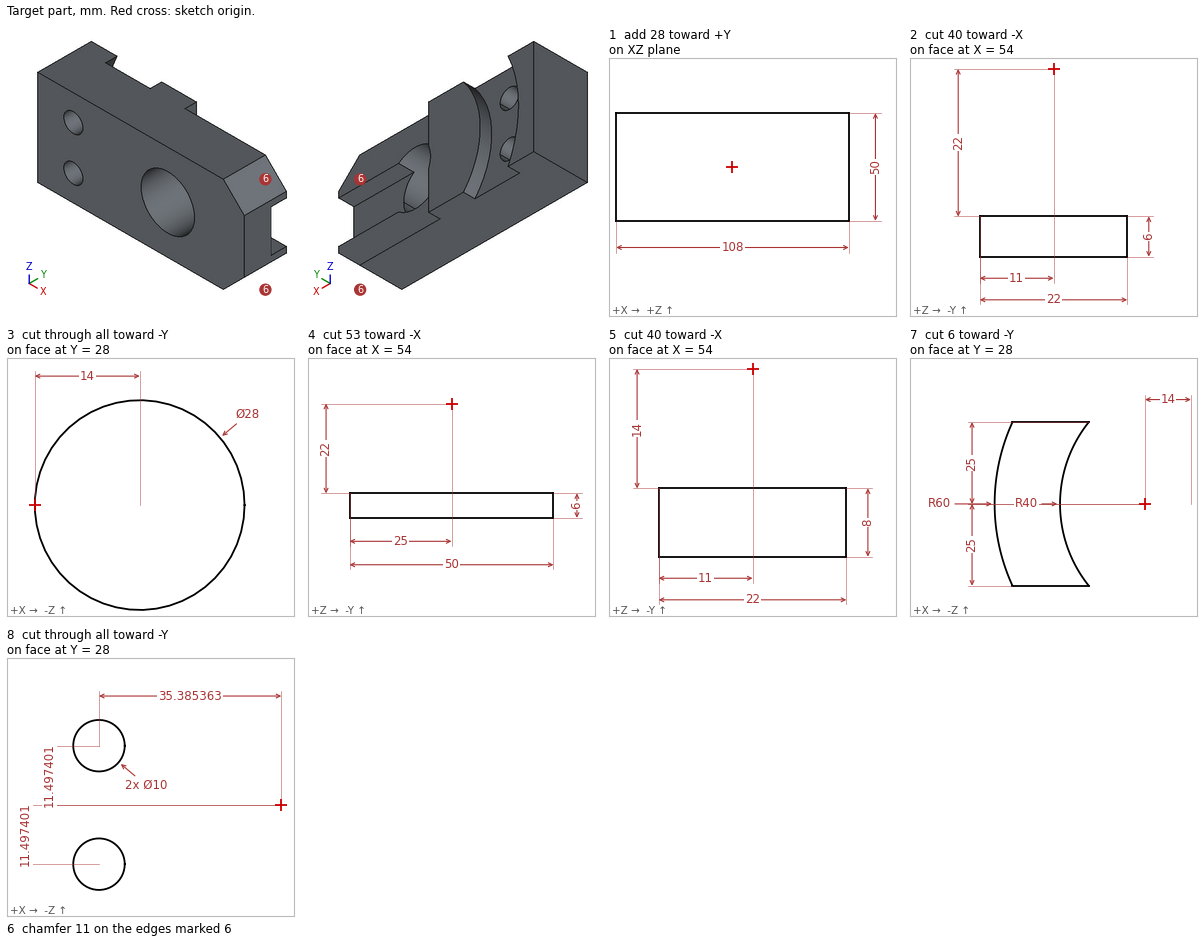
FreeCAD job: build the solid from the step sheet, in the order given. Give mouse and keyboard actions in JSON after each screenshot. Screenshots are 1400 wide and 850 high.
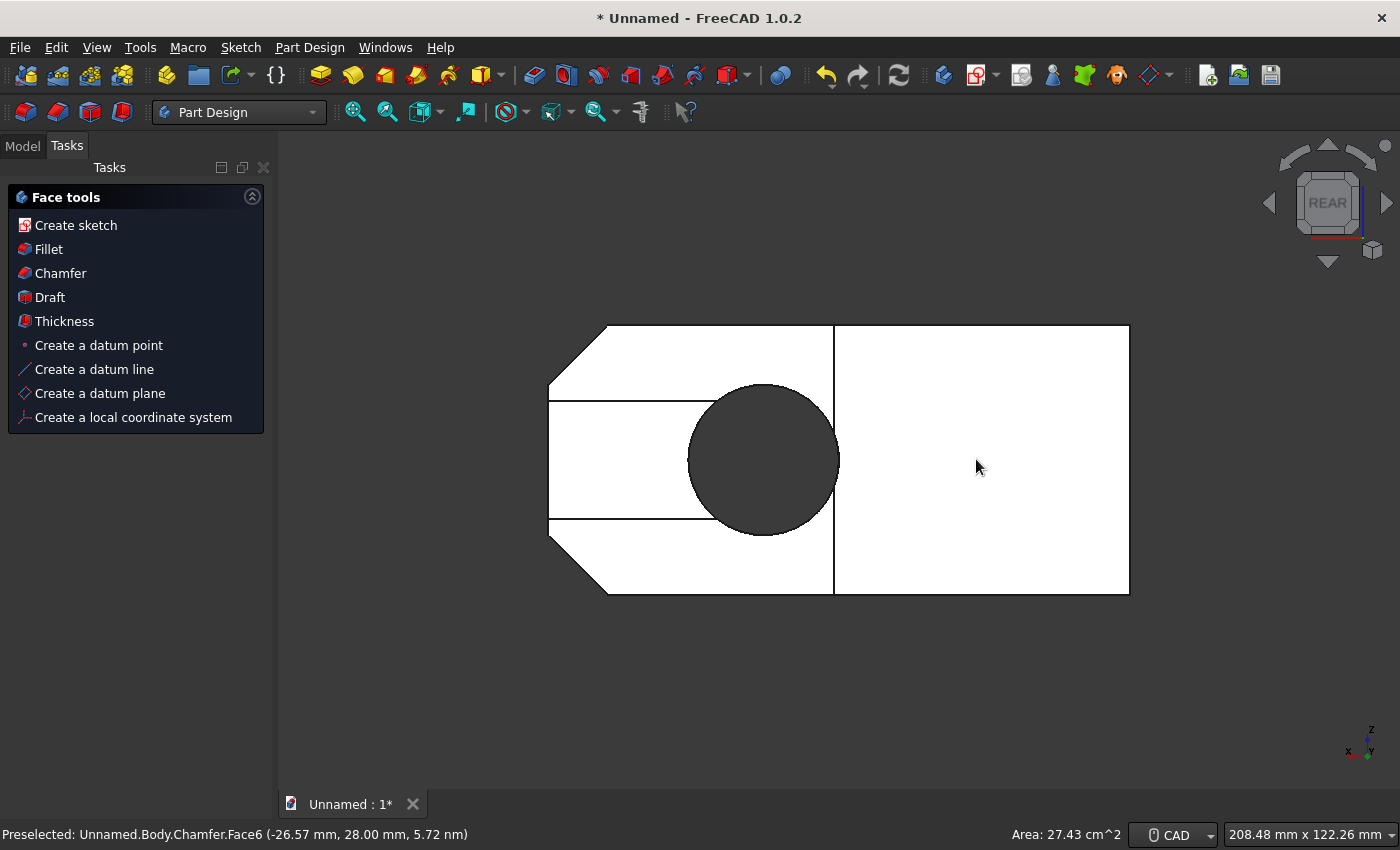
{"action": "left_click", "coordinate": [976, 76]}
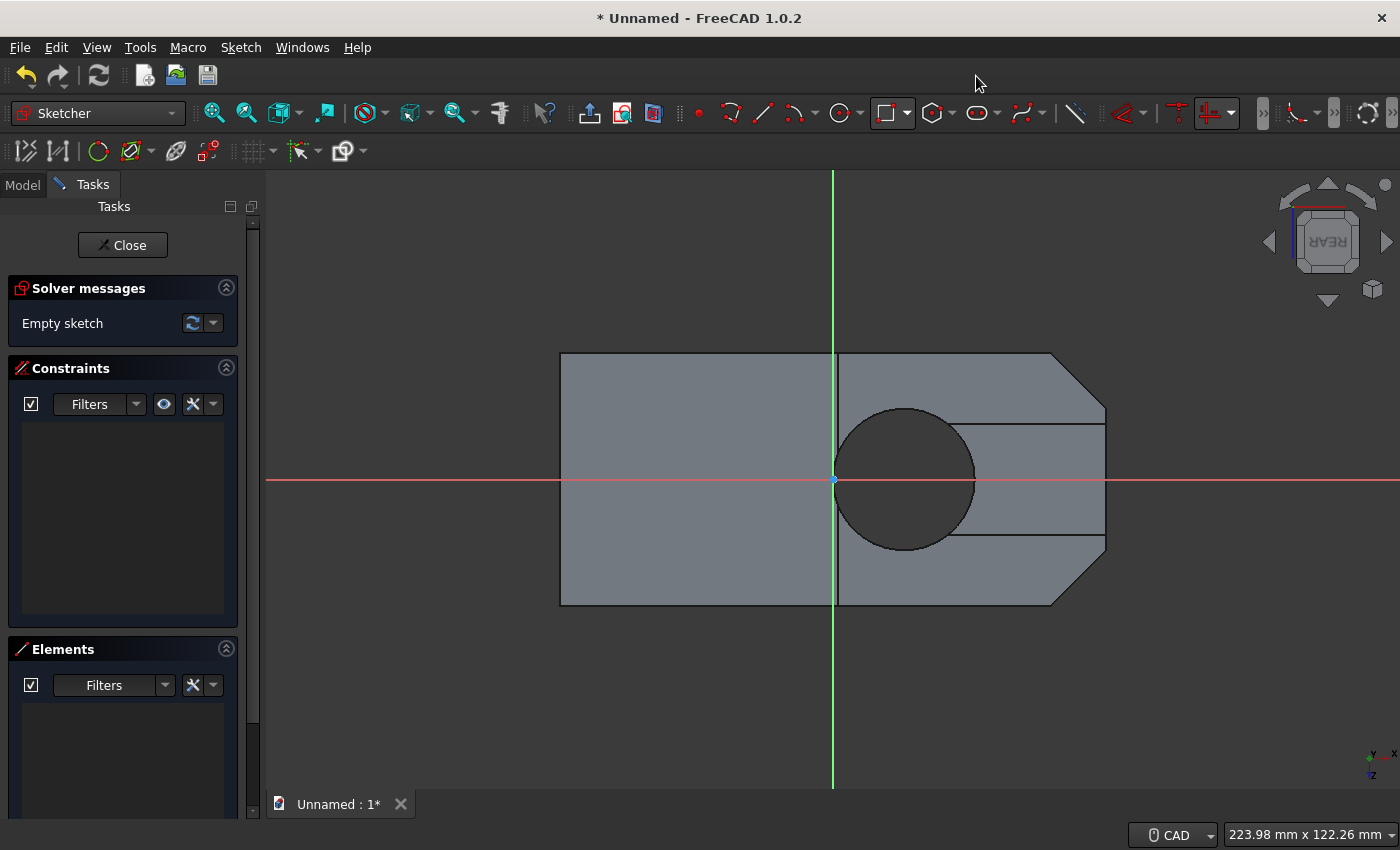
{"action": "scroll", "coordinate": [619, 479], "scroll_direction": "up", "scroll_amount": 2}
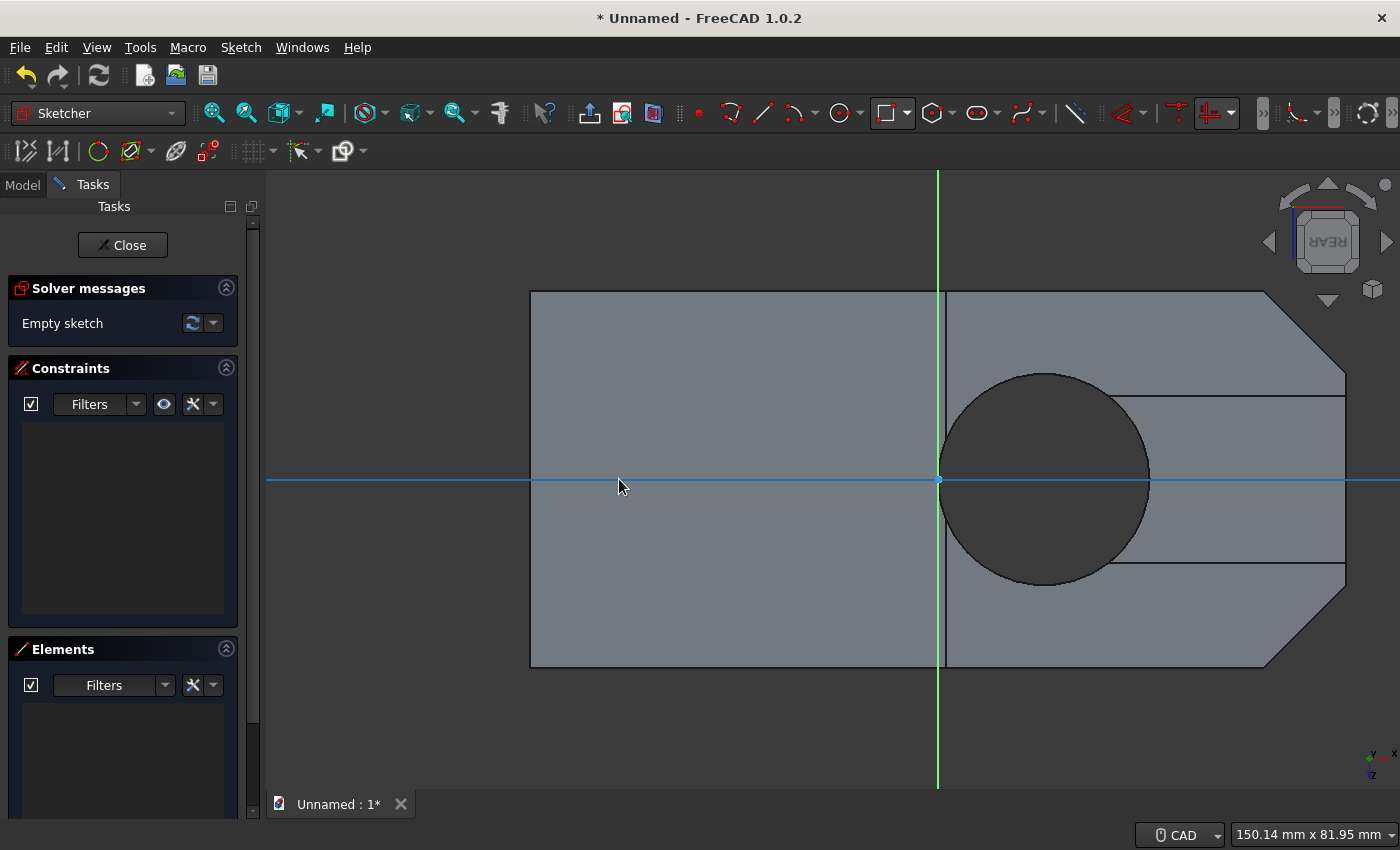
{"action": "key", "text": "g l"}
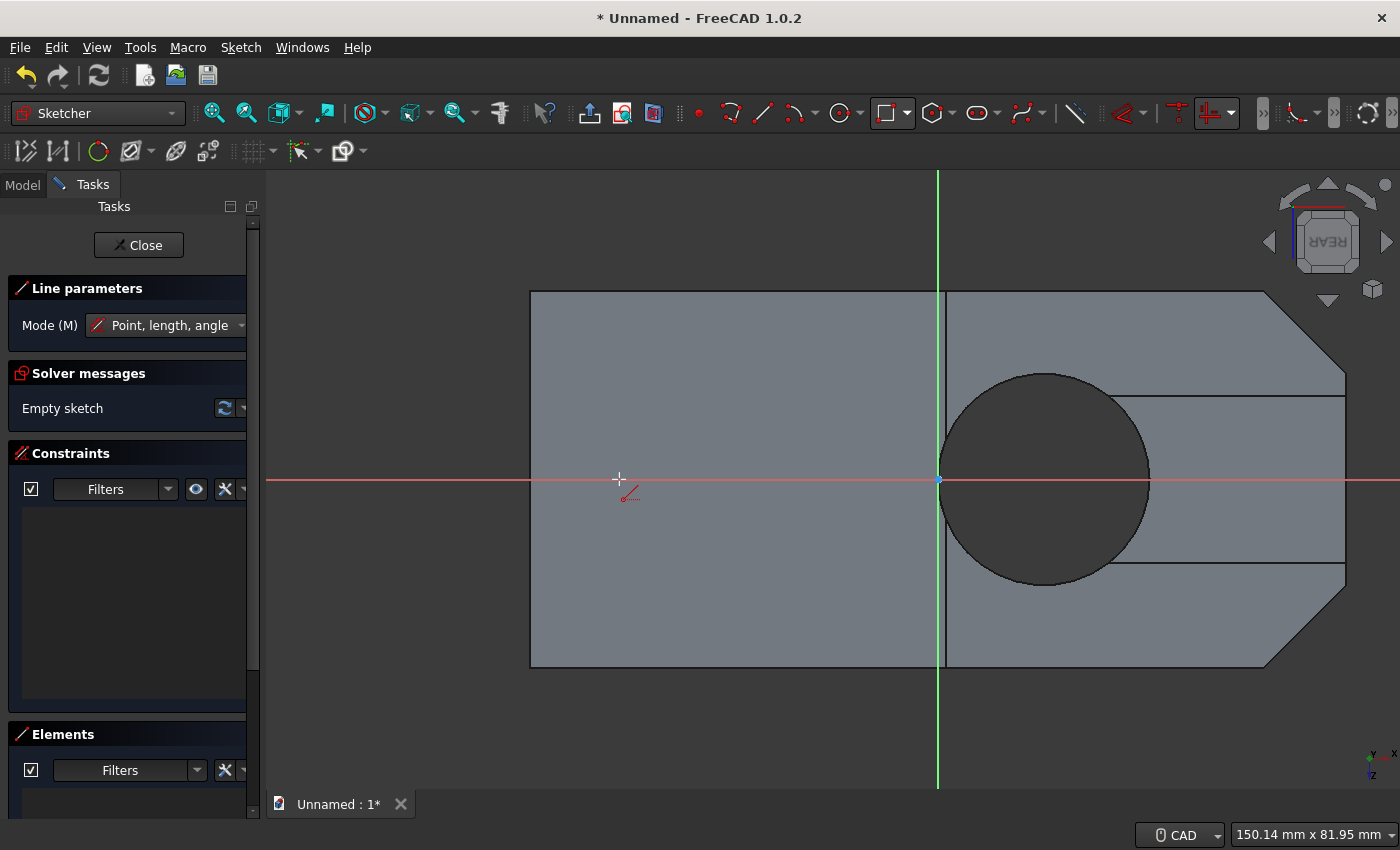
{"action": "left_click", "coordinate": [632, 668]}
{"action": "left_click", "coordinate": [808, 668]}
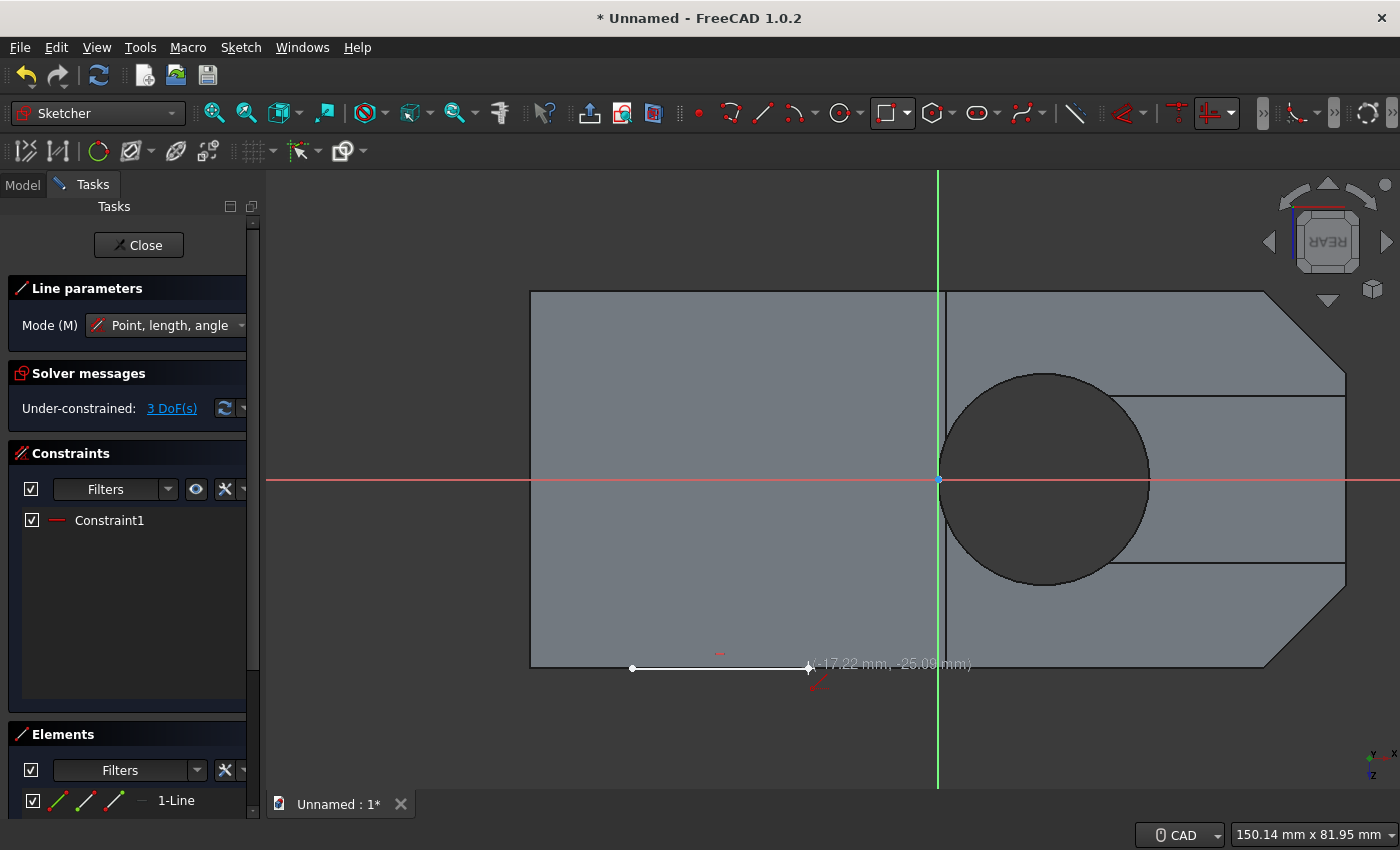
{"action": "left_click", "coordinate": [808, 291]}
{"action": "left_click", "coordinate": [632, 291]}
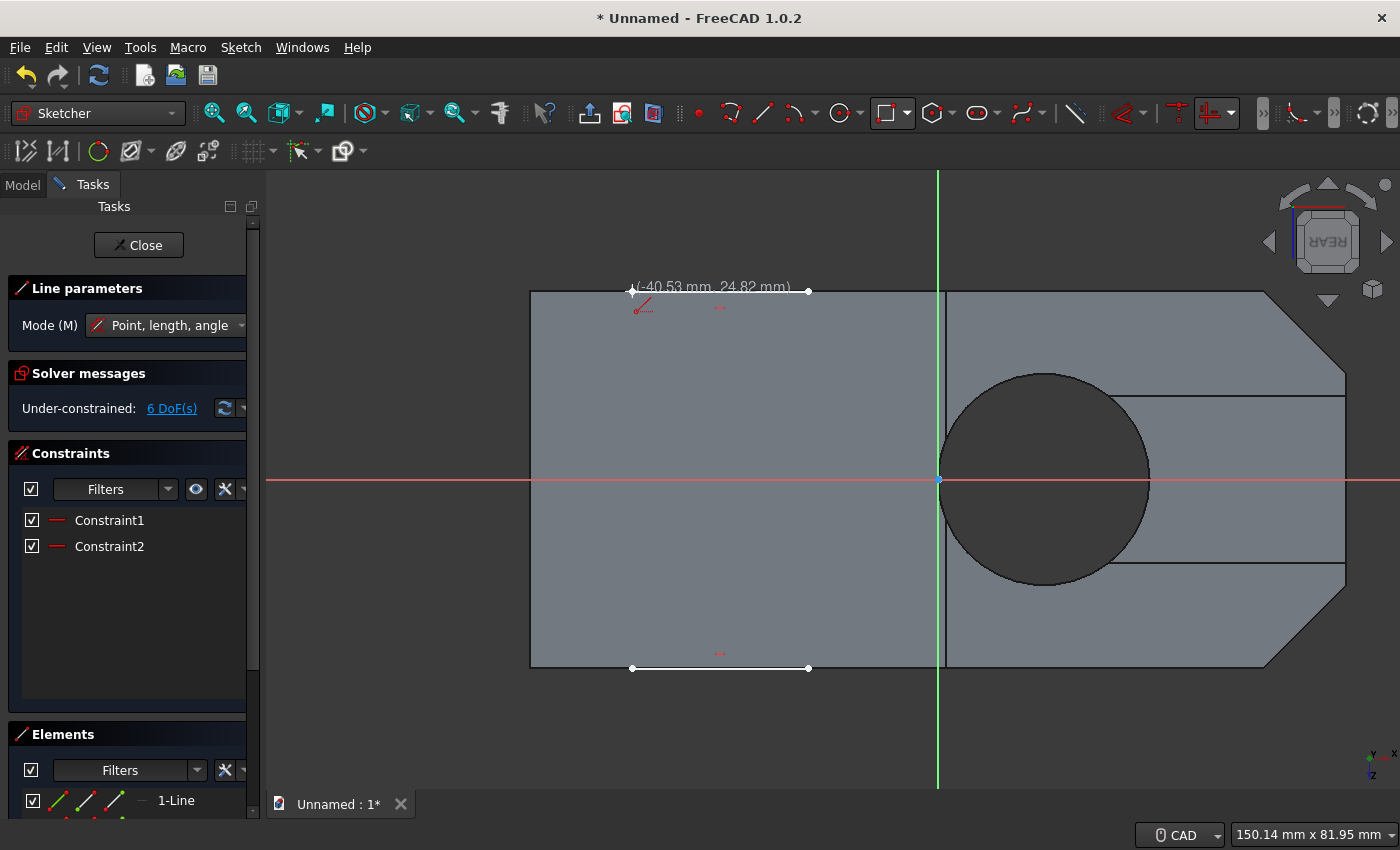
{"action": "key", "text": "g 3 a"}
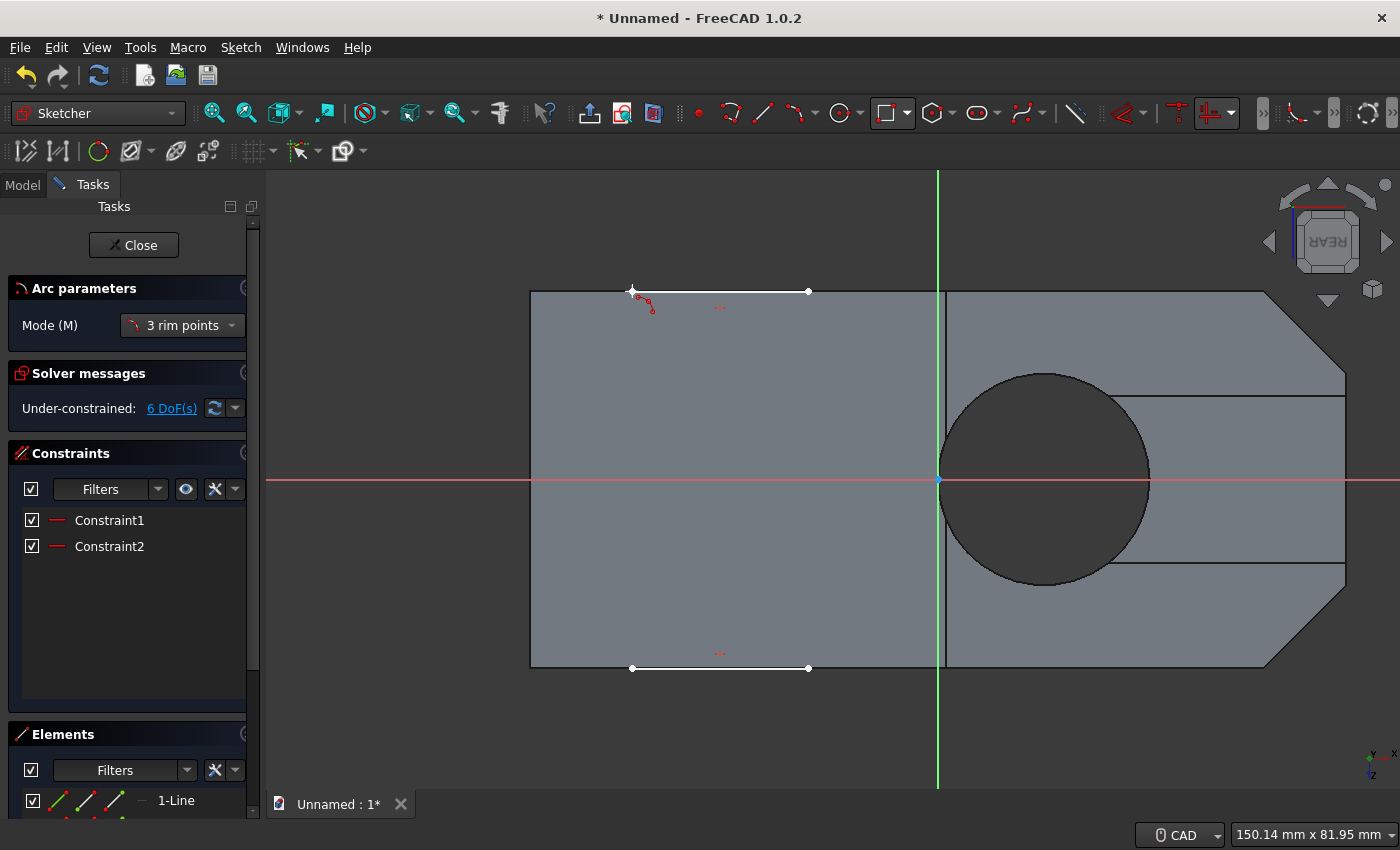
{"action": "left_click", "coordinate": [808, 669]}
{"action": "left_click", "coordinate": [808, 292]}
{"action": "left_click", "coordinate": [744, 439]}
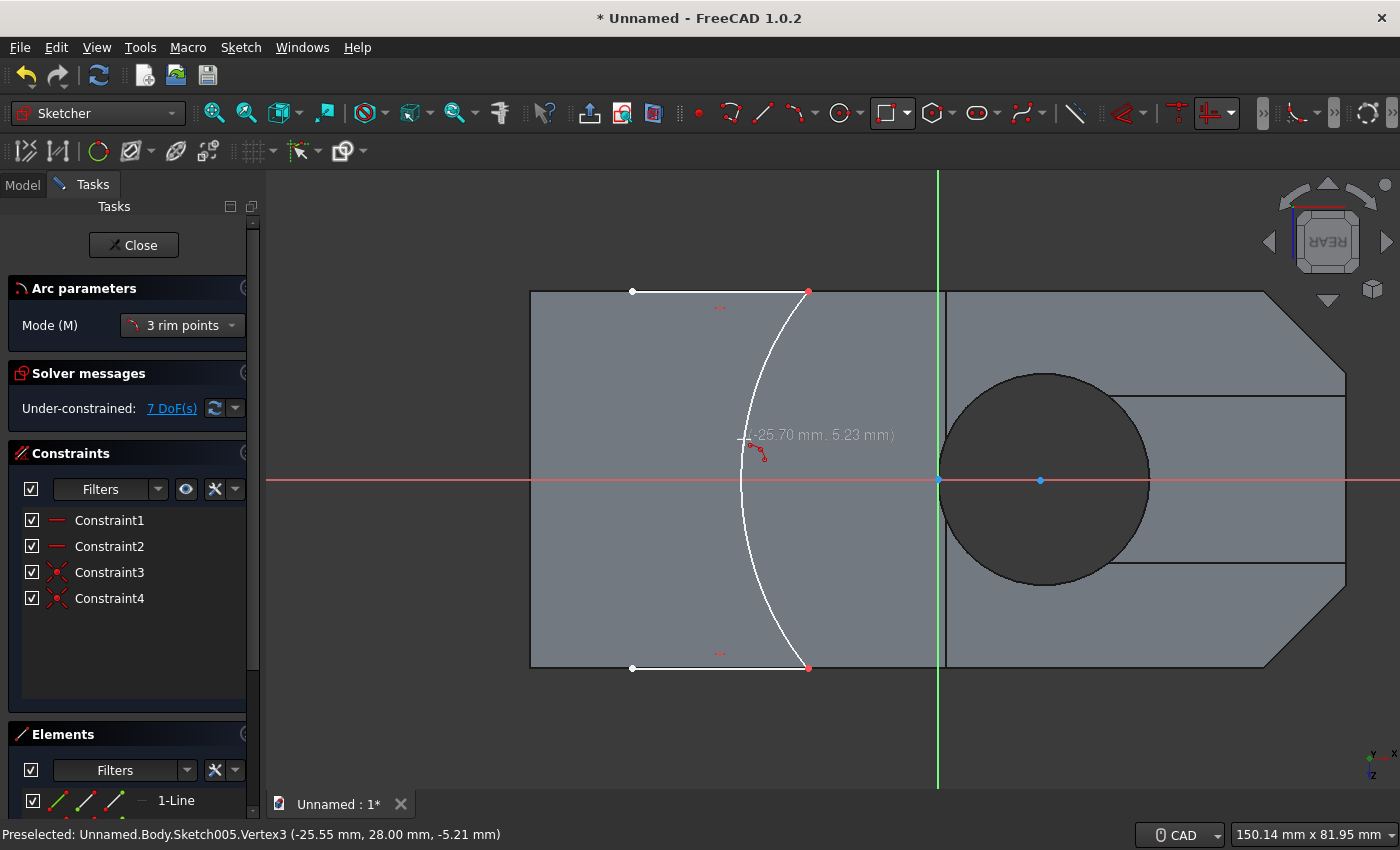
{"action": "left_click", "coordinate": [632, 292]}
{"action": "left_click", "coordinate": [632, 669]}
{"action": "left_click", "coordinate": [592, 441]}
{"action": "key", "text": "Escape"}